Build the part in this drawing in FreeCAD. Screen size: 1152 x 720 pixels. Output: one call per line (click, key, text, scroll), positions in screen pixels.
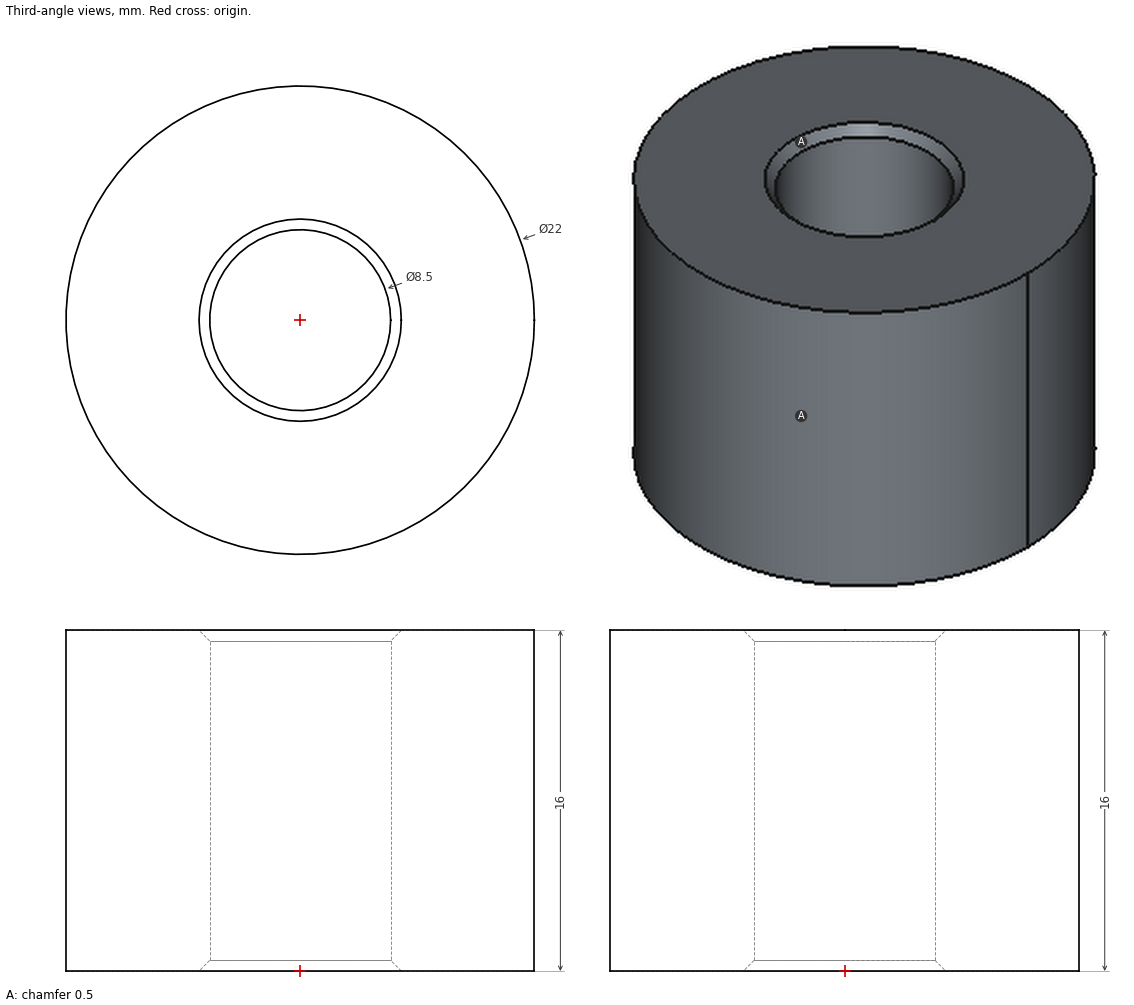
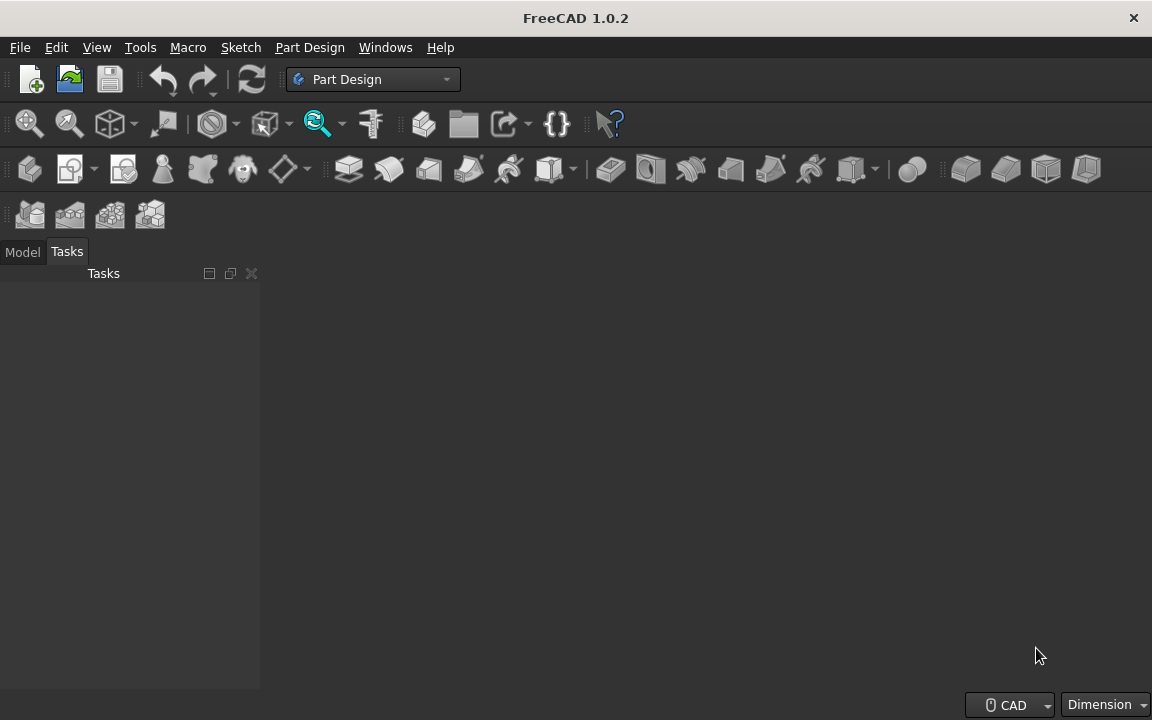
click(30, 80)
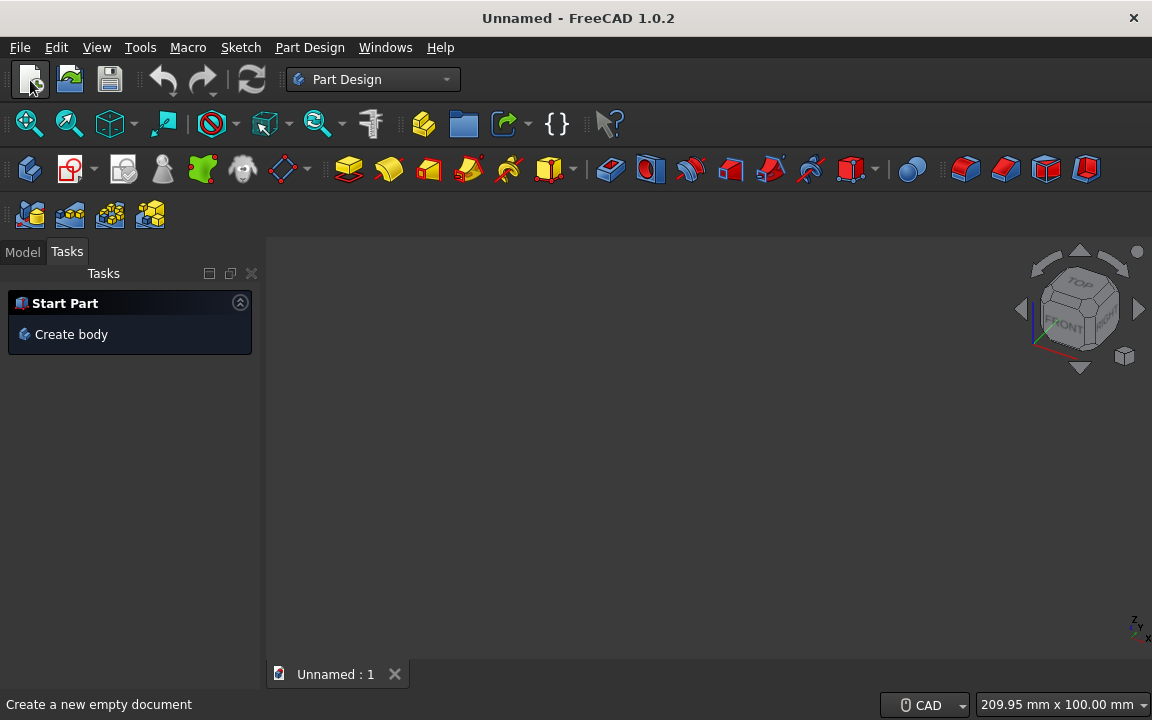
click(70, 170)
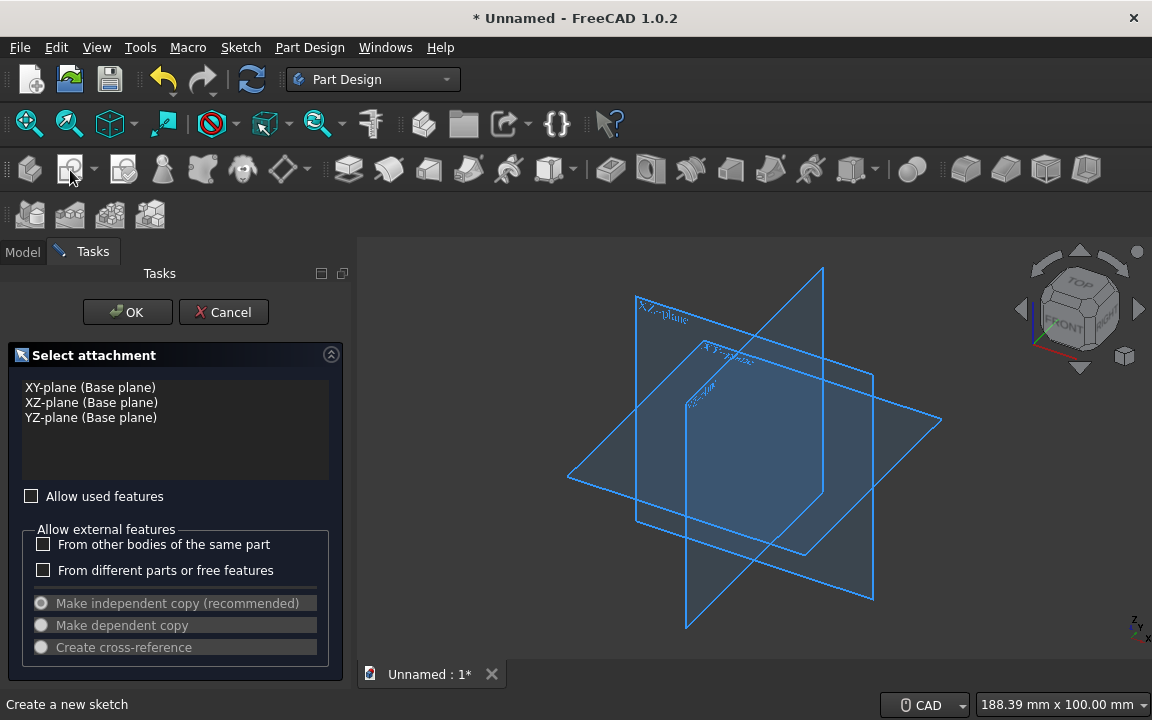
click(82, 388)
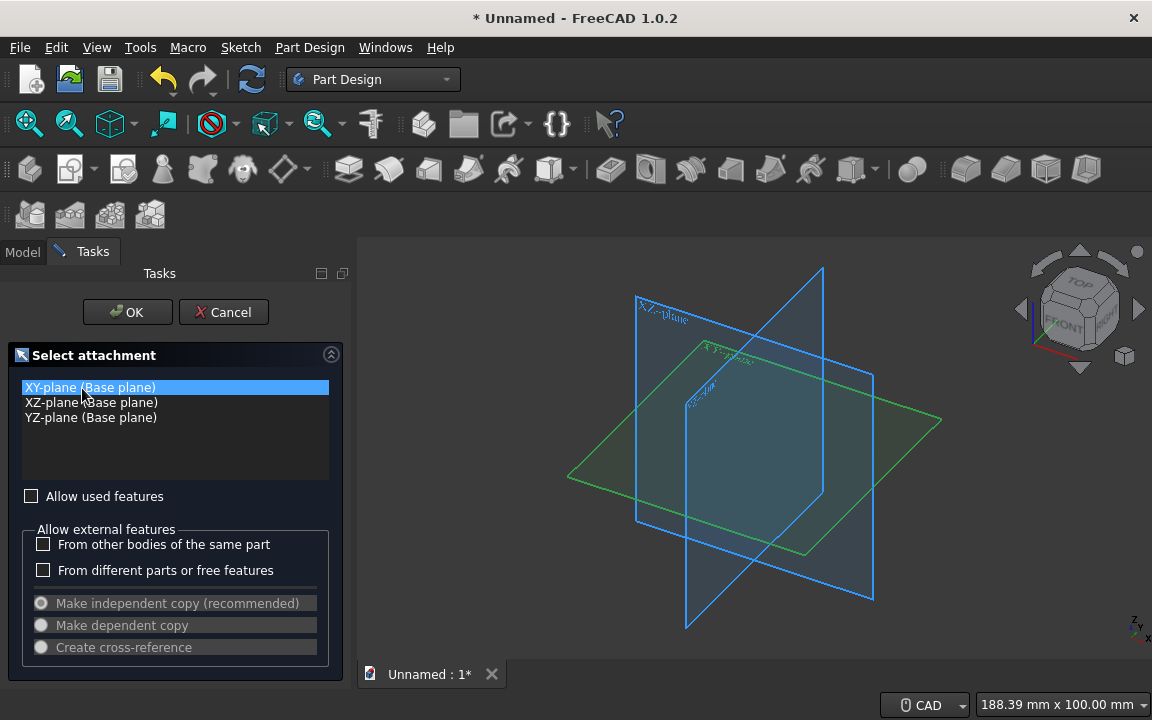
click(128, 312)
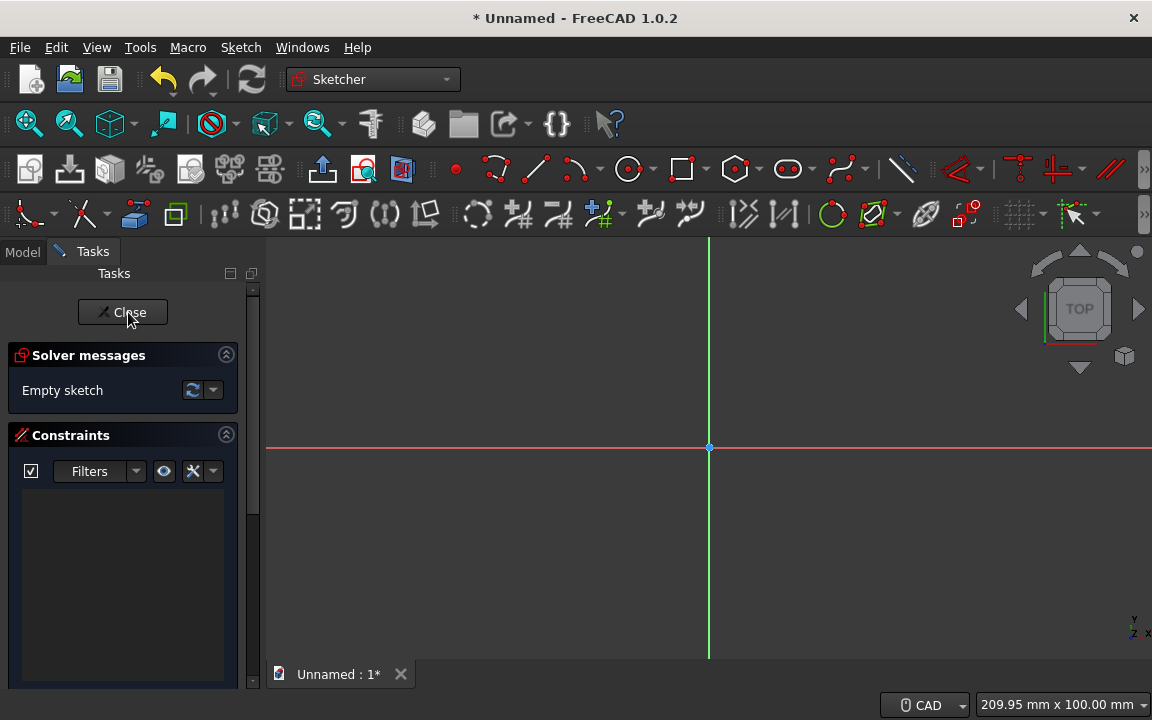
scroll(749, 448, up, 5)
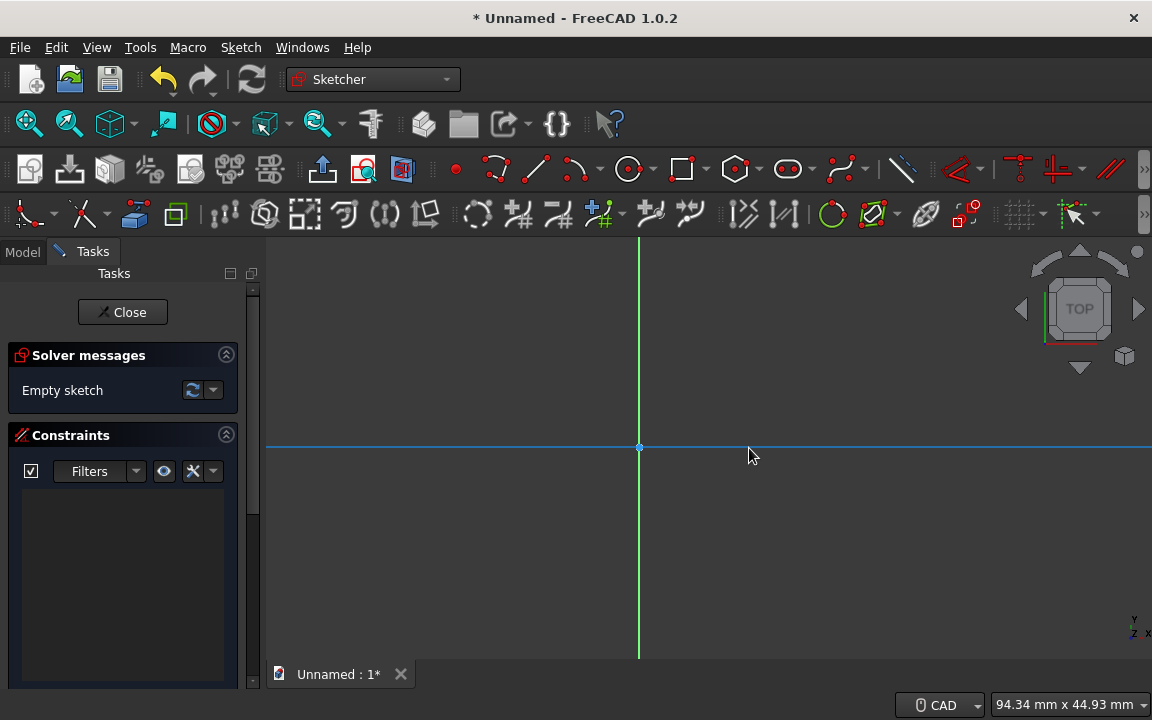
click(630, 170)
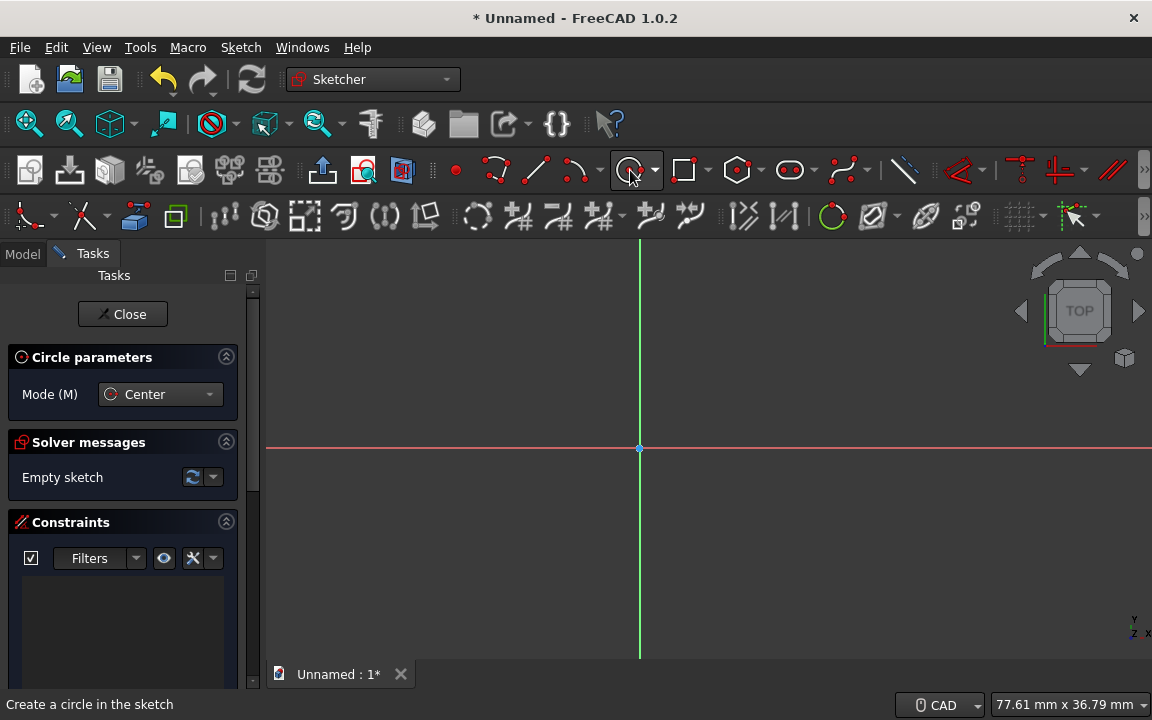
click(640, 448)
click(728, 359)
key(Escape)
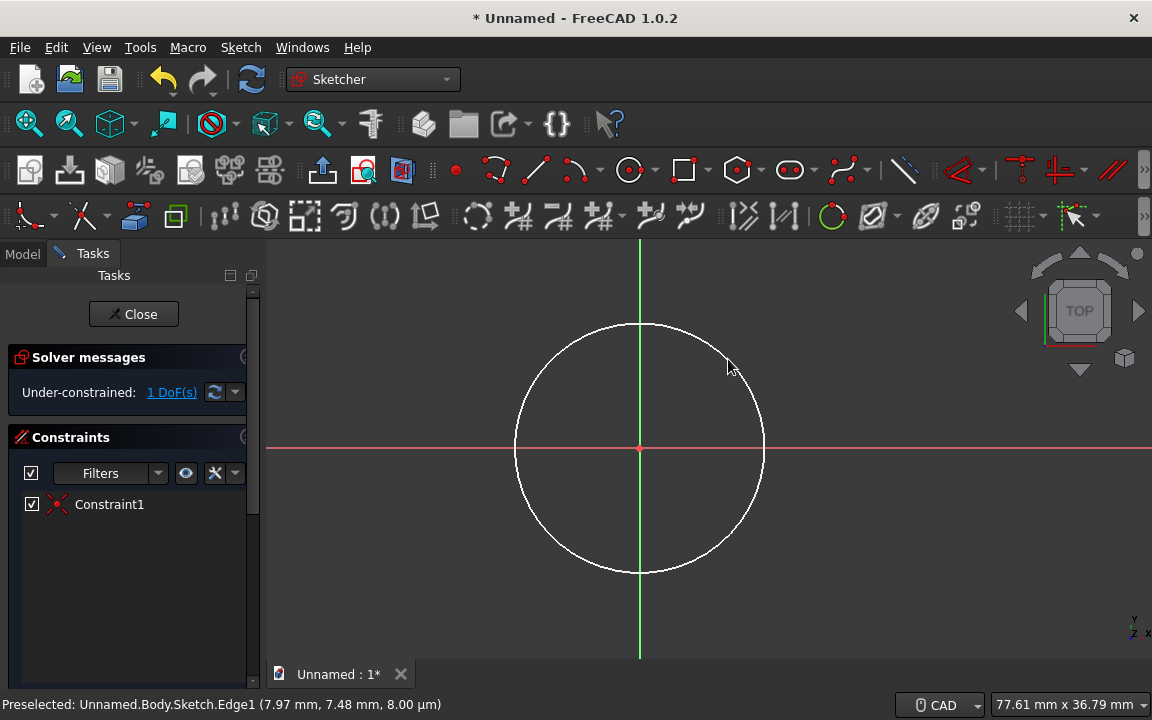
click(958, 170)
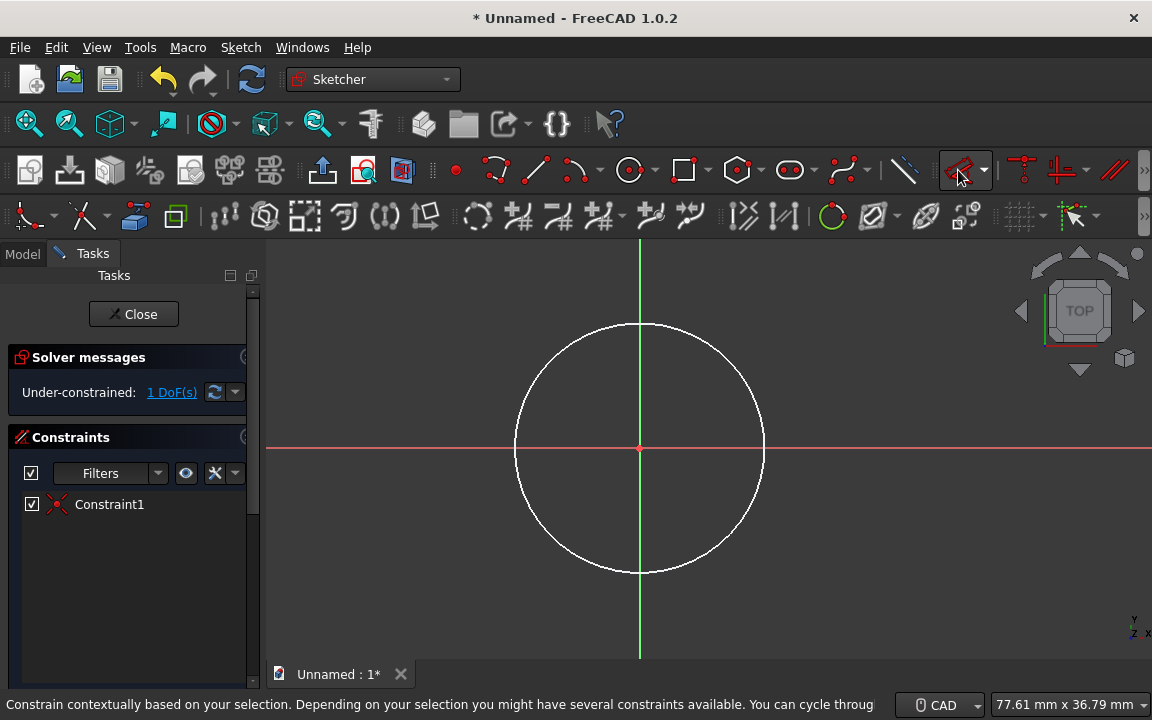
click(728, 360)
click(751, 337)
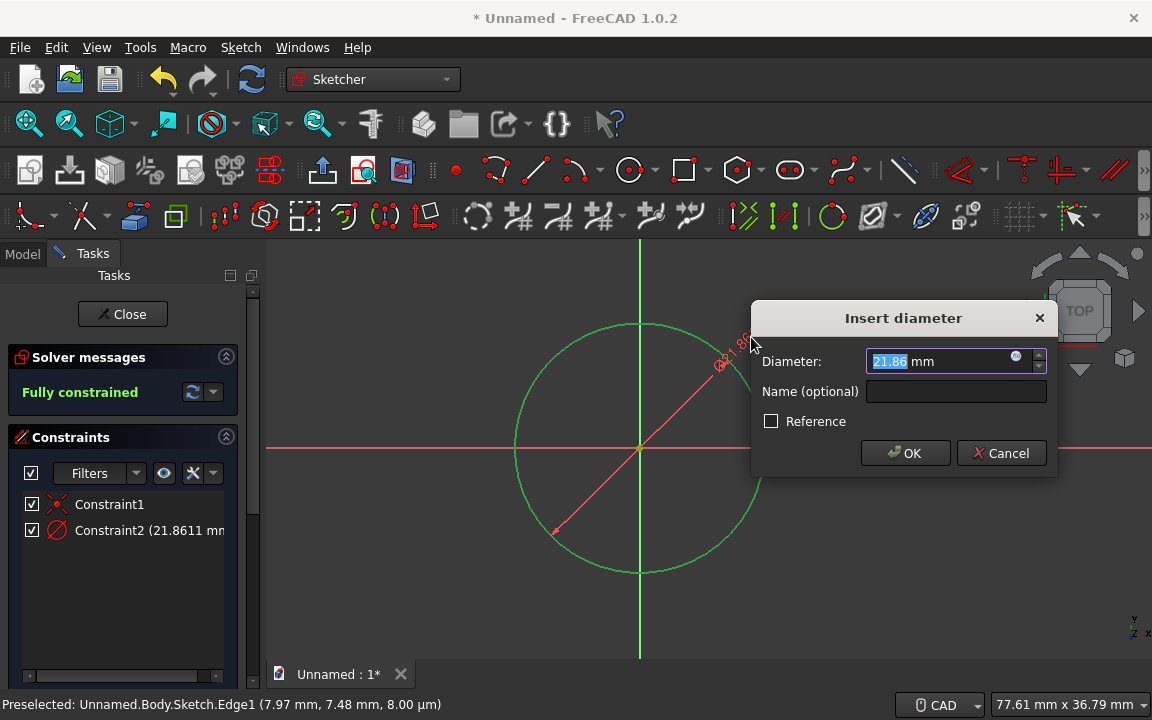
text(22)
key(Return)
key(Escape)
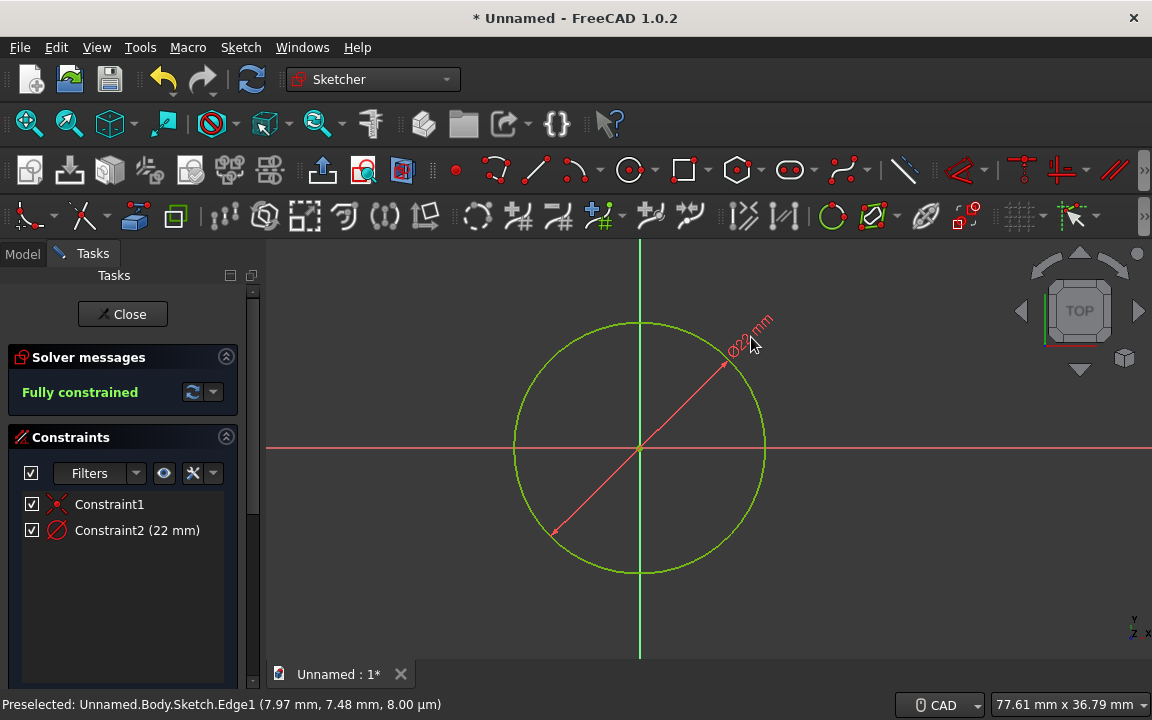
click(123, 314)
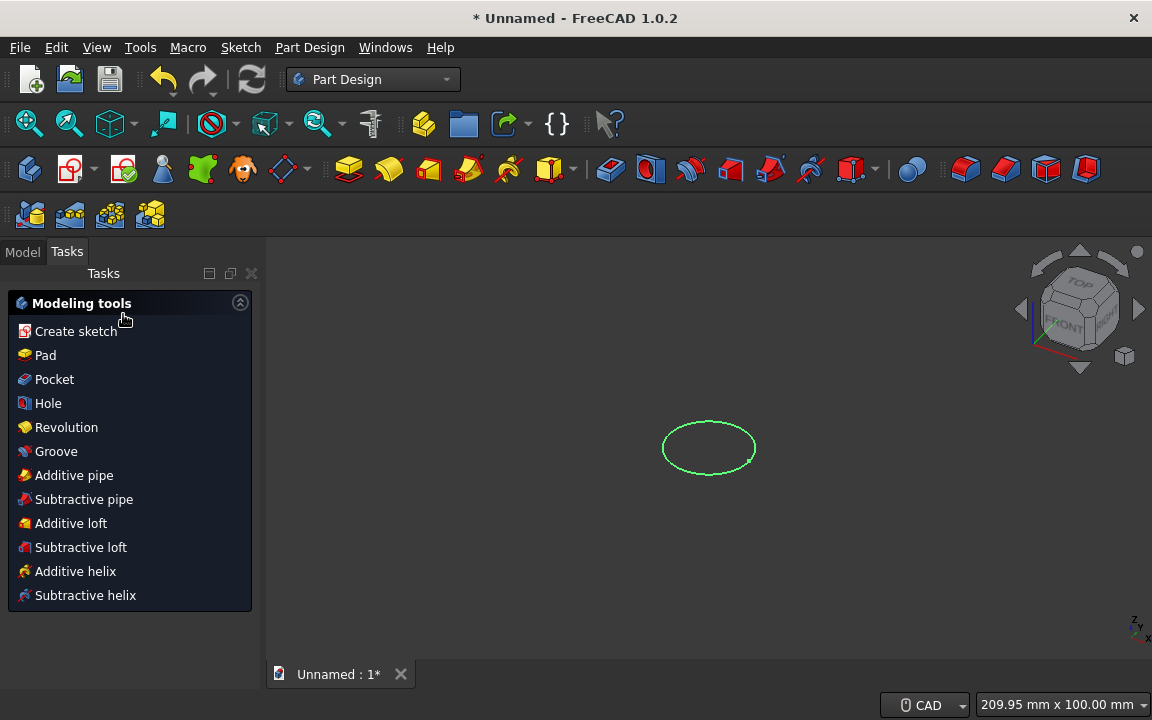
click(350, 170)